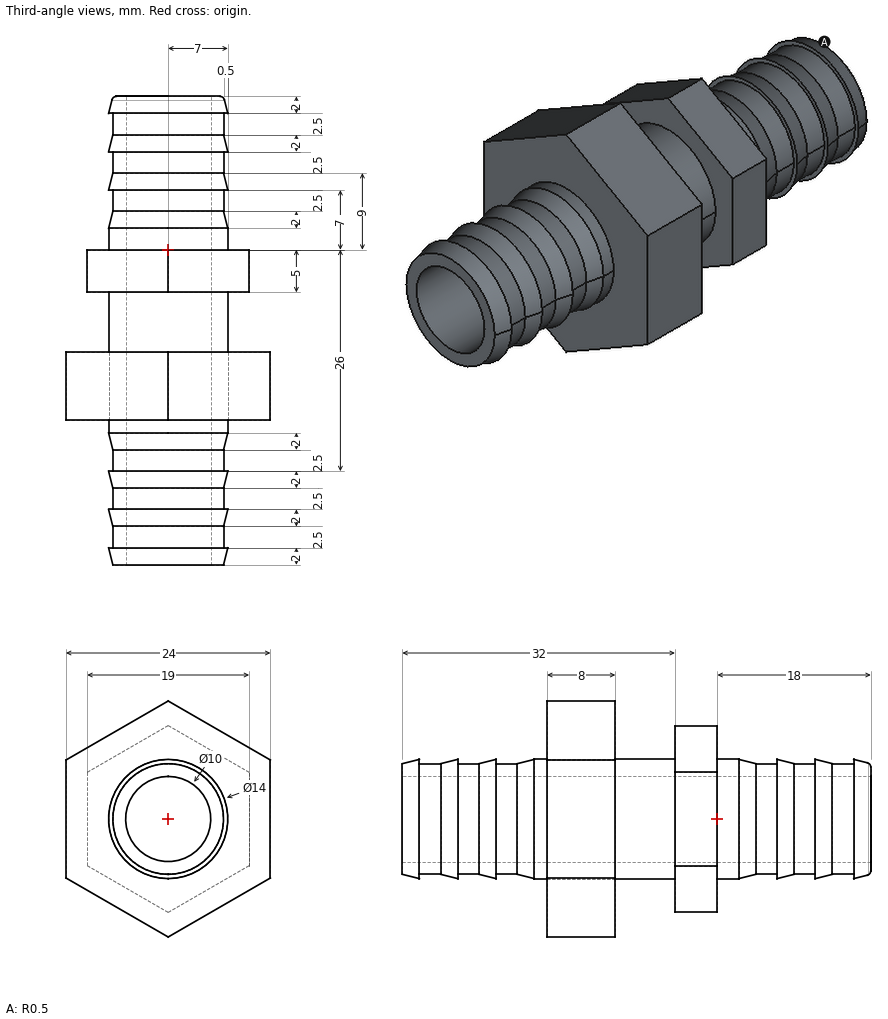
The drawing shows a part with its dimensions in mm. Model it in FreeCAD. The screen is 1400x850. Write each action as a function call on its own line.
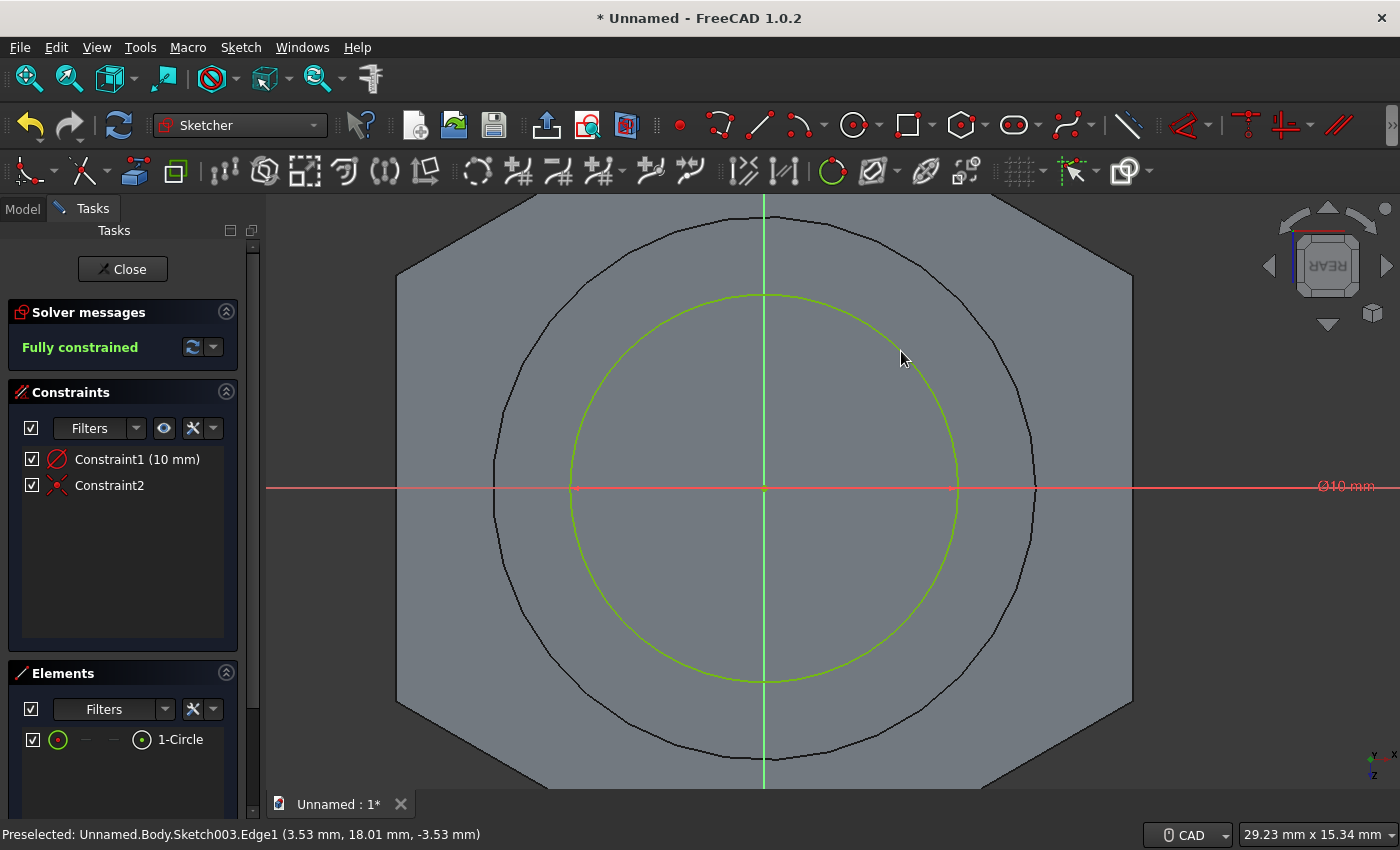
click(123, 269)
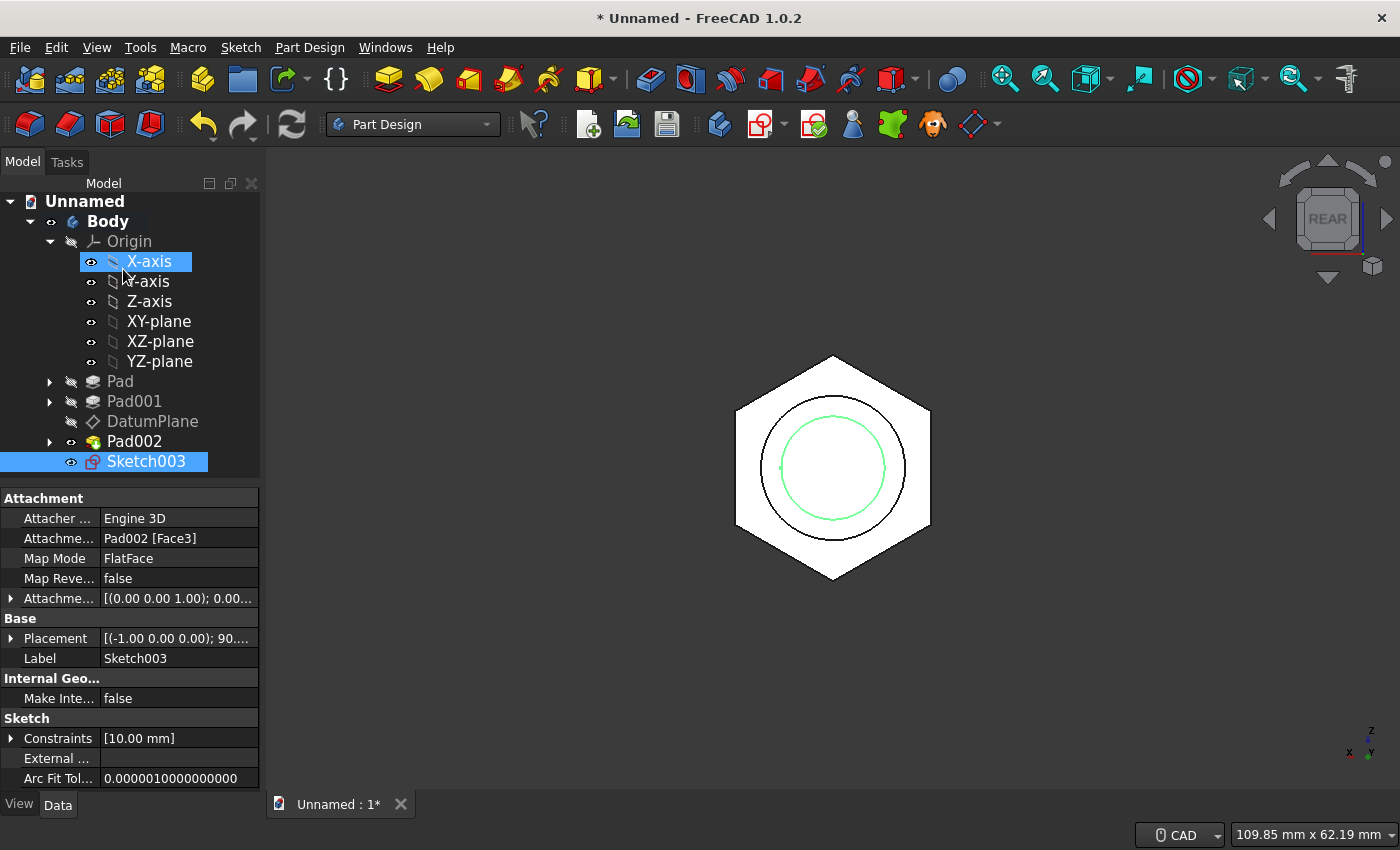
click(652, 80)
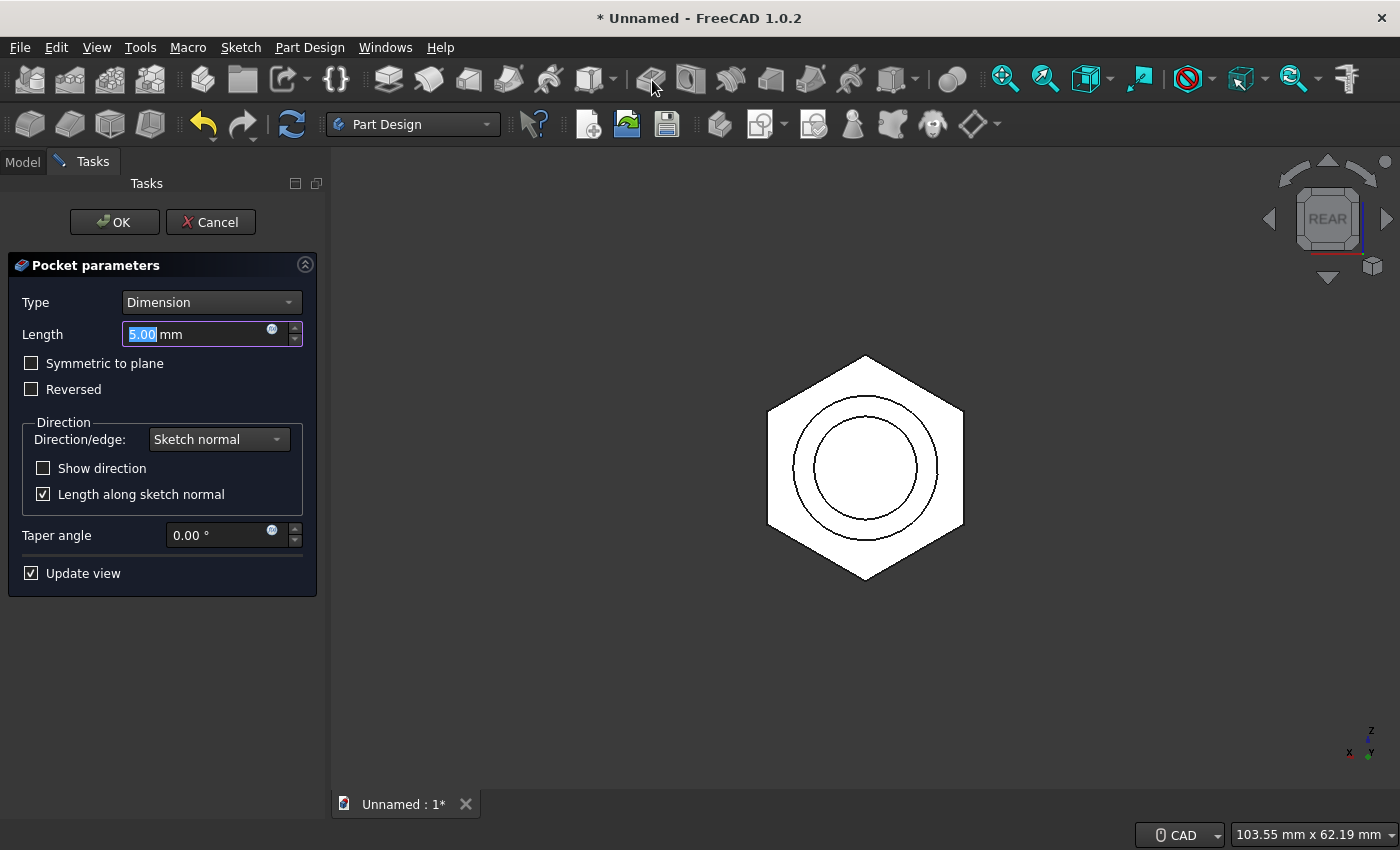
click(212, 302)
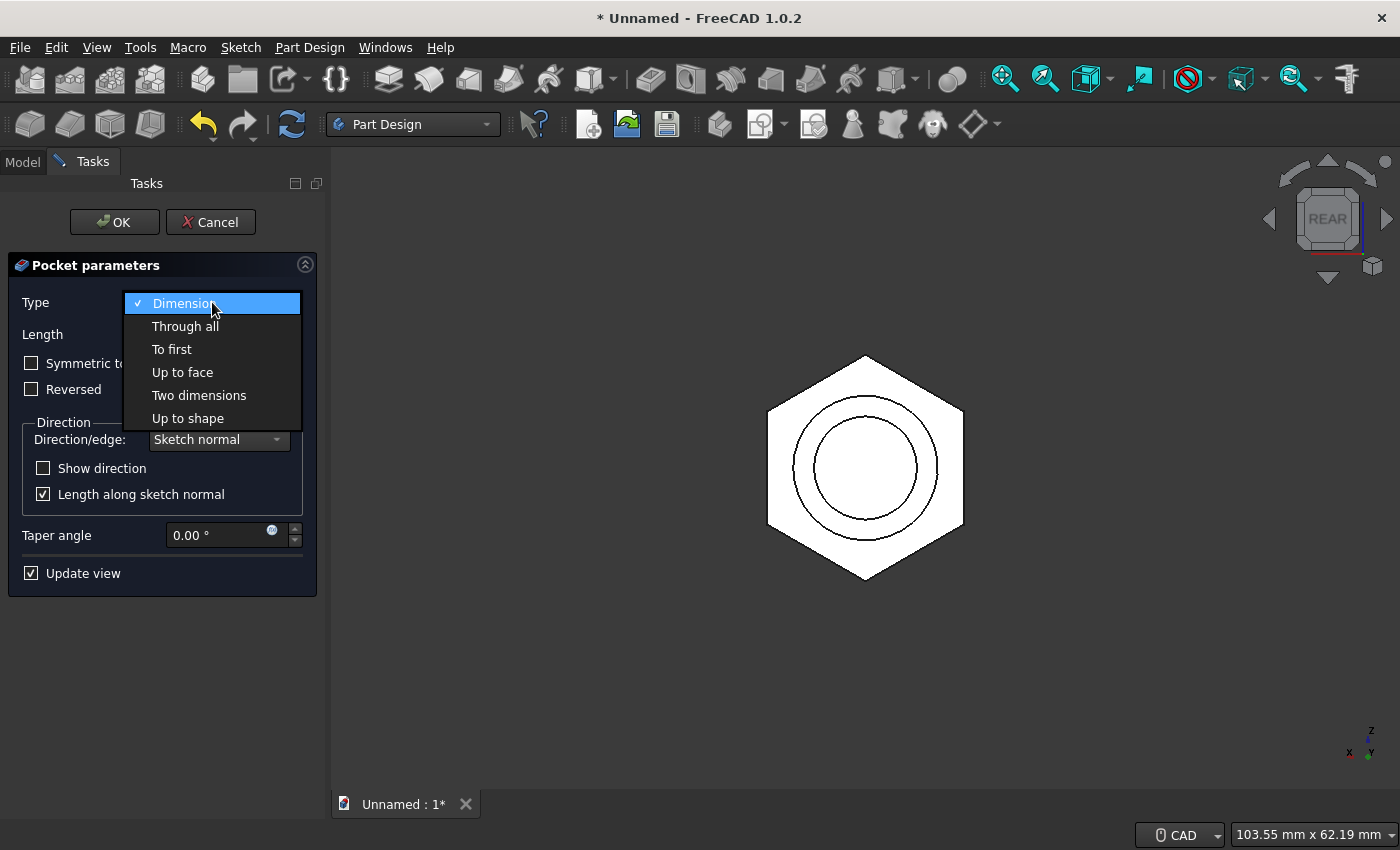
click(212, 326)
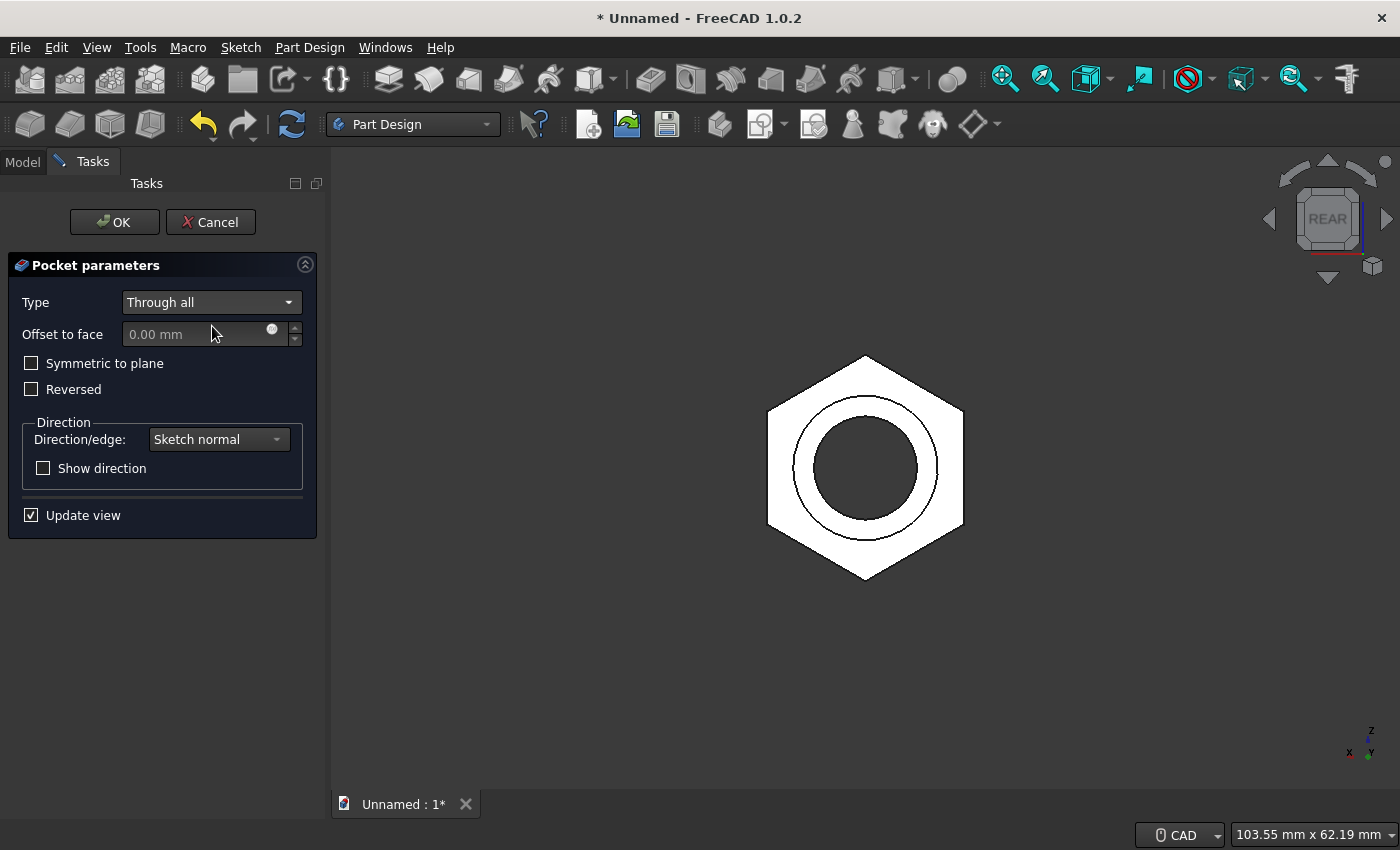
click(115, 222)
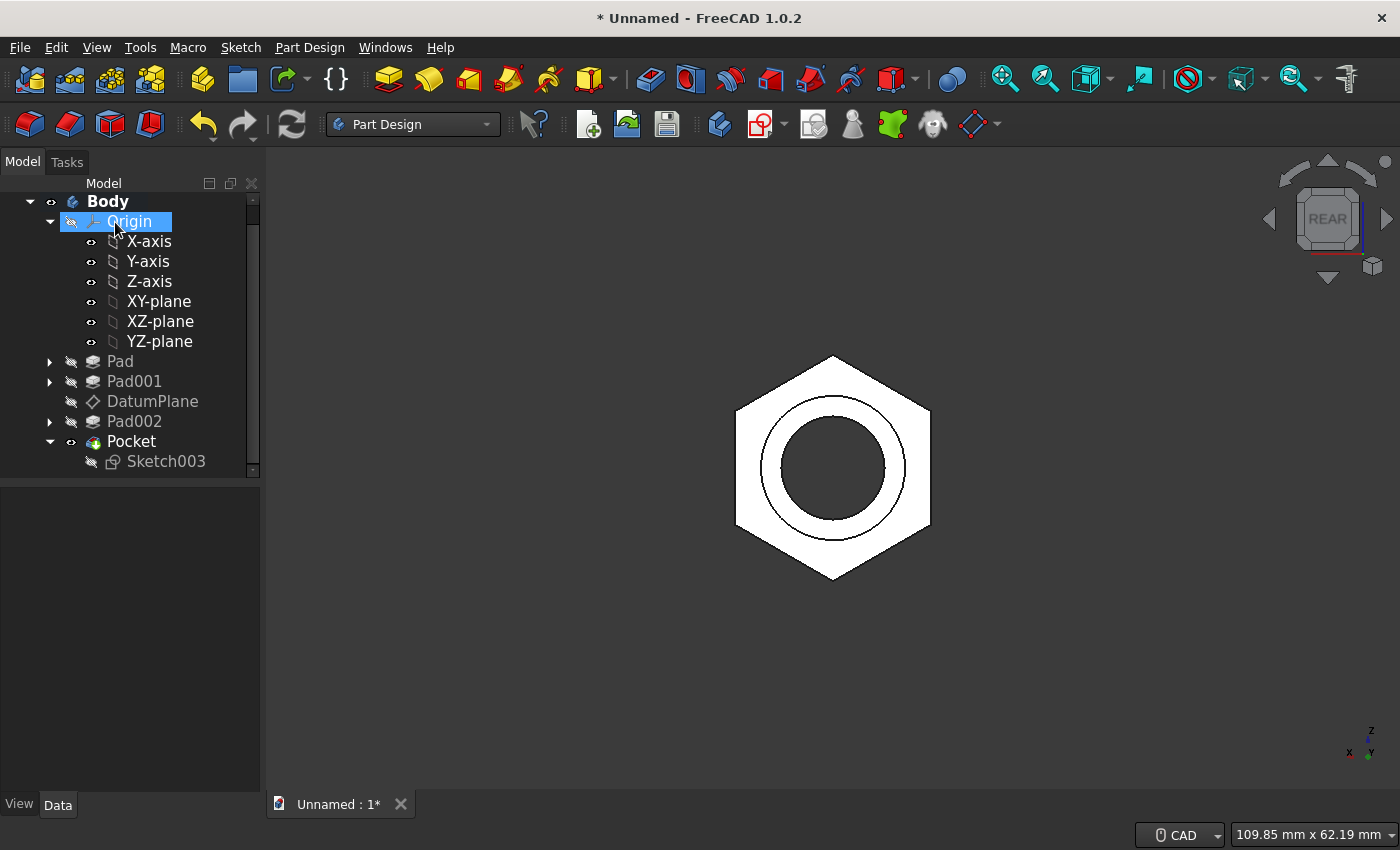
click(1006, 80)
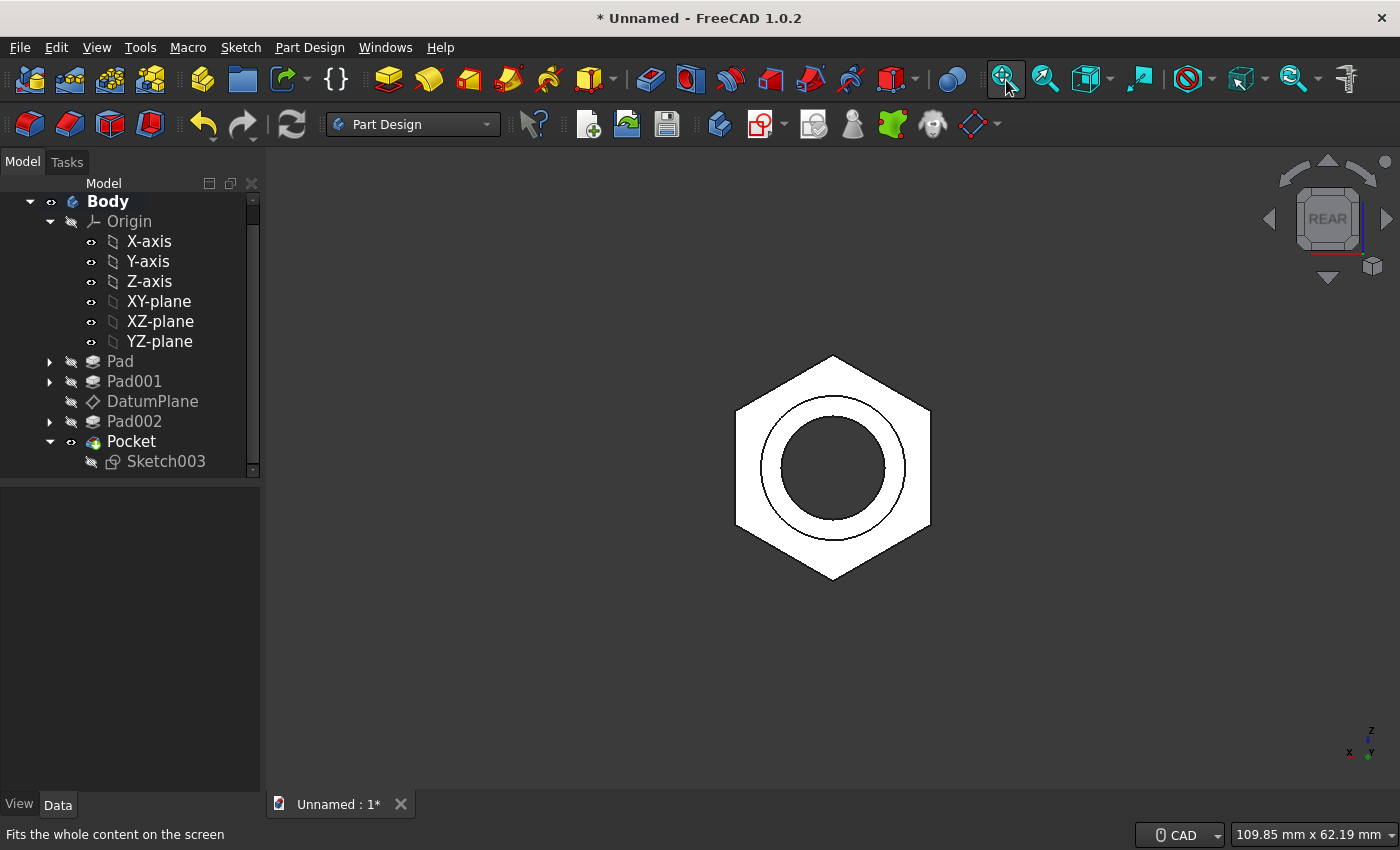
click(760, 124)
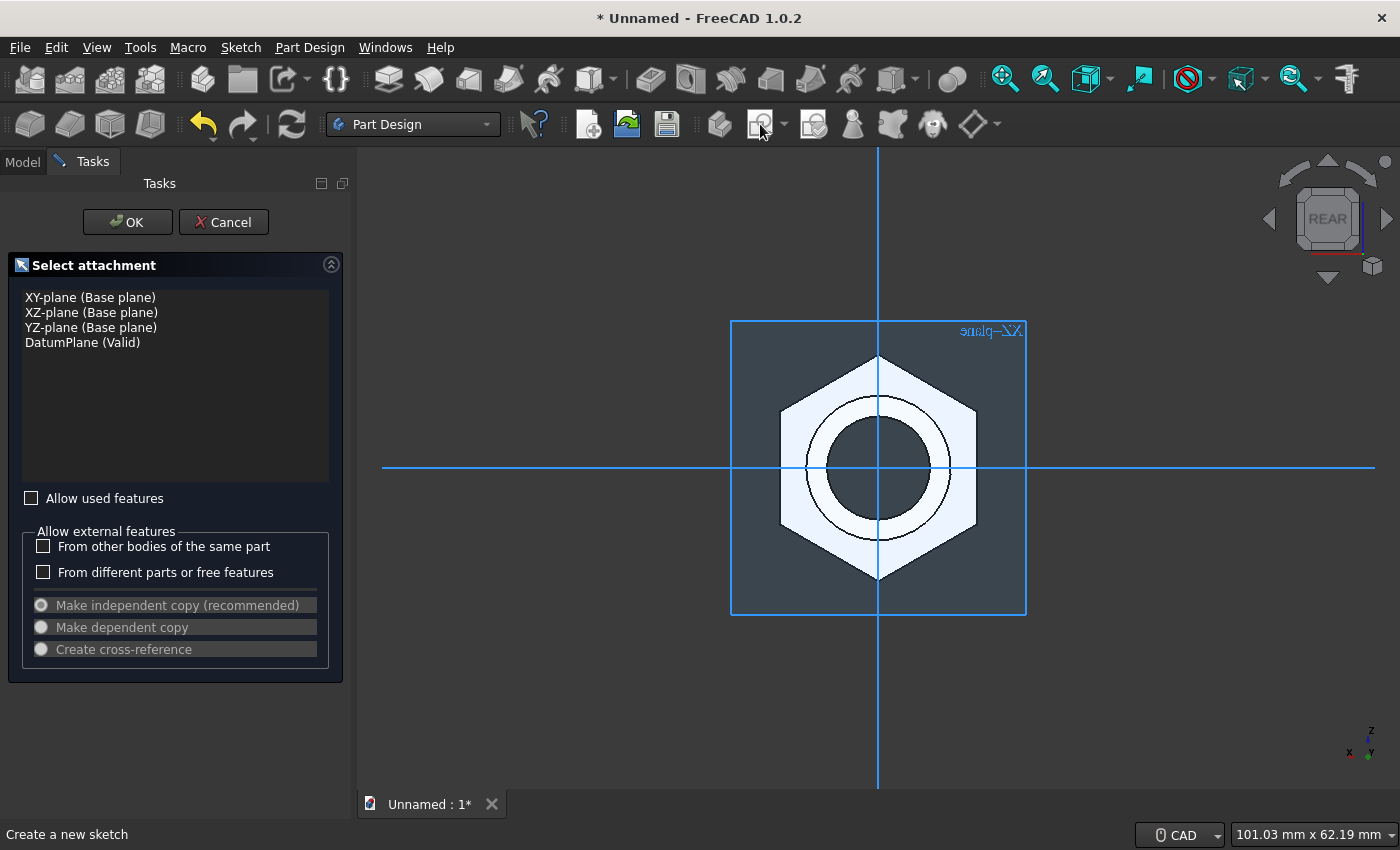
click(82, 298)